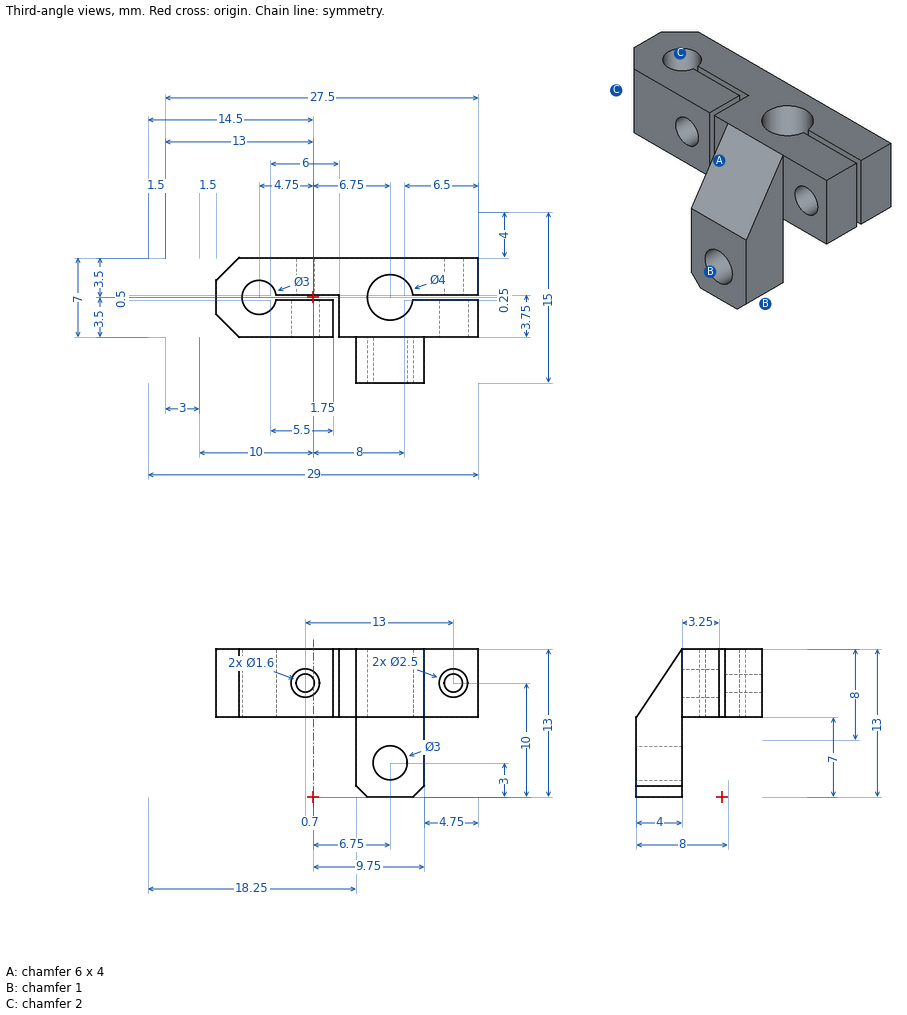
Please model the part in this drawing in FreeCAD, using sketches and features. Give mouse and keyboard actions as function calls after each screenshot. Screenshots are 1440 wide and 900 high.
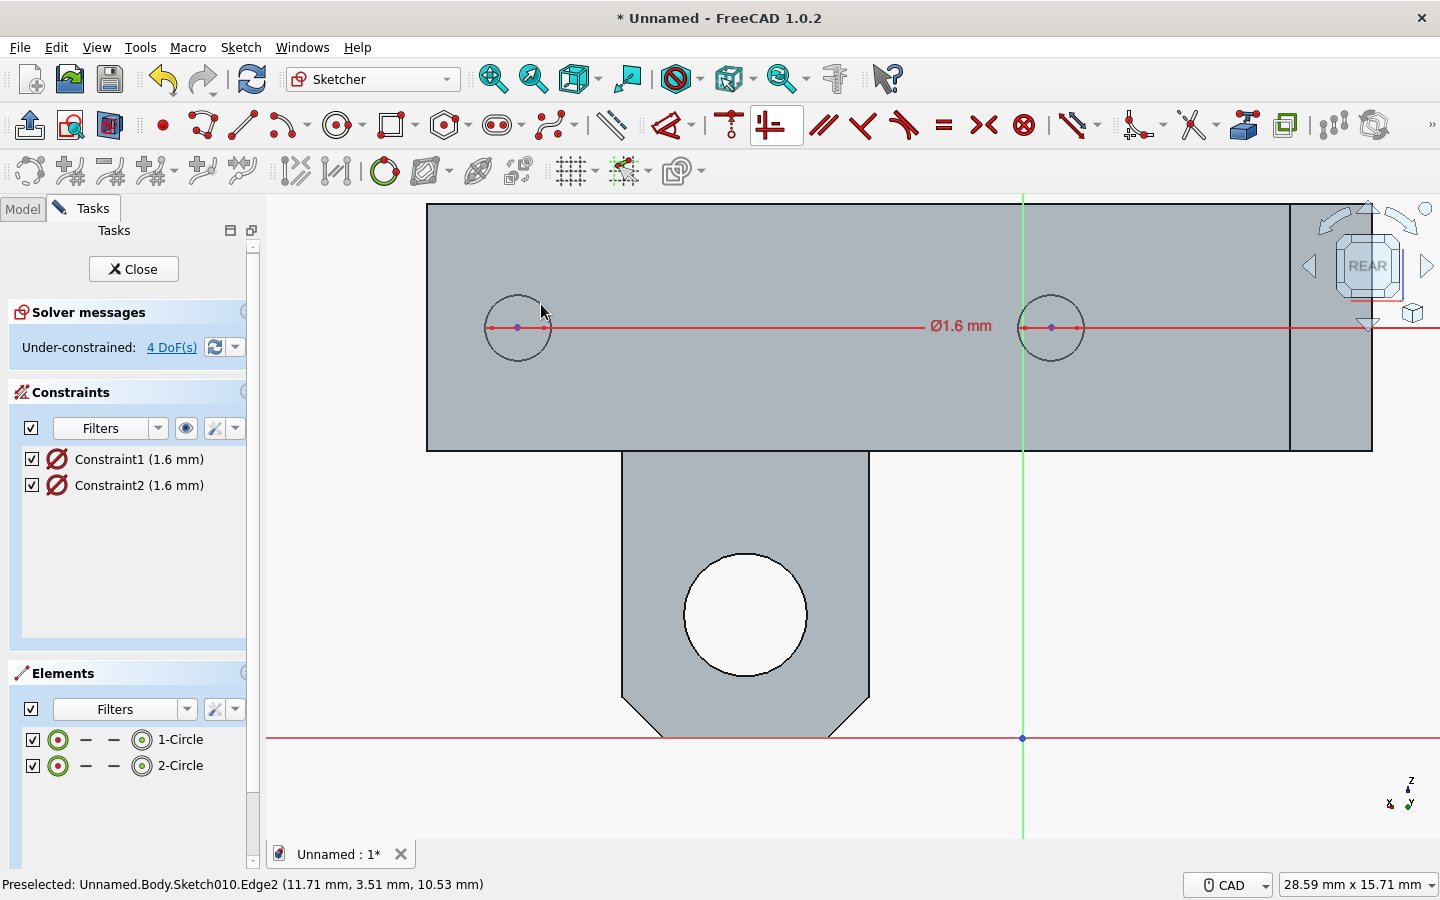
click(1051, 328)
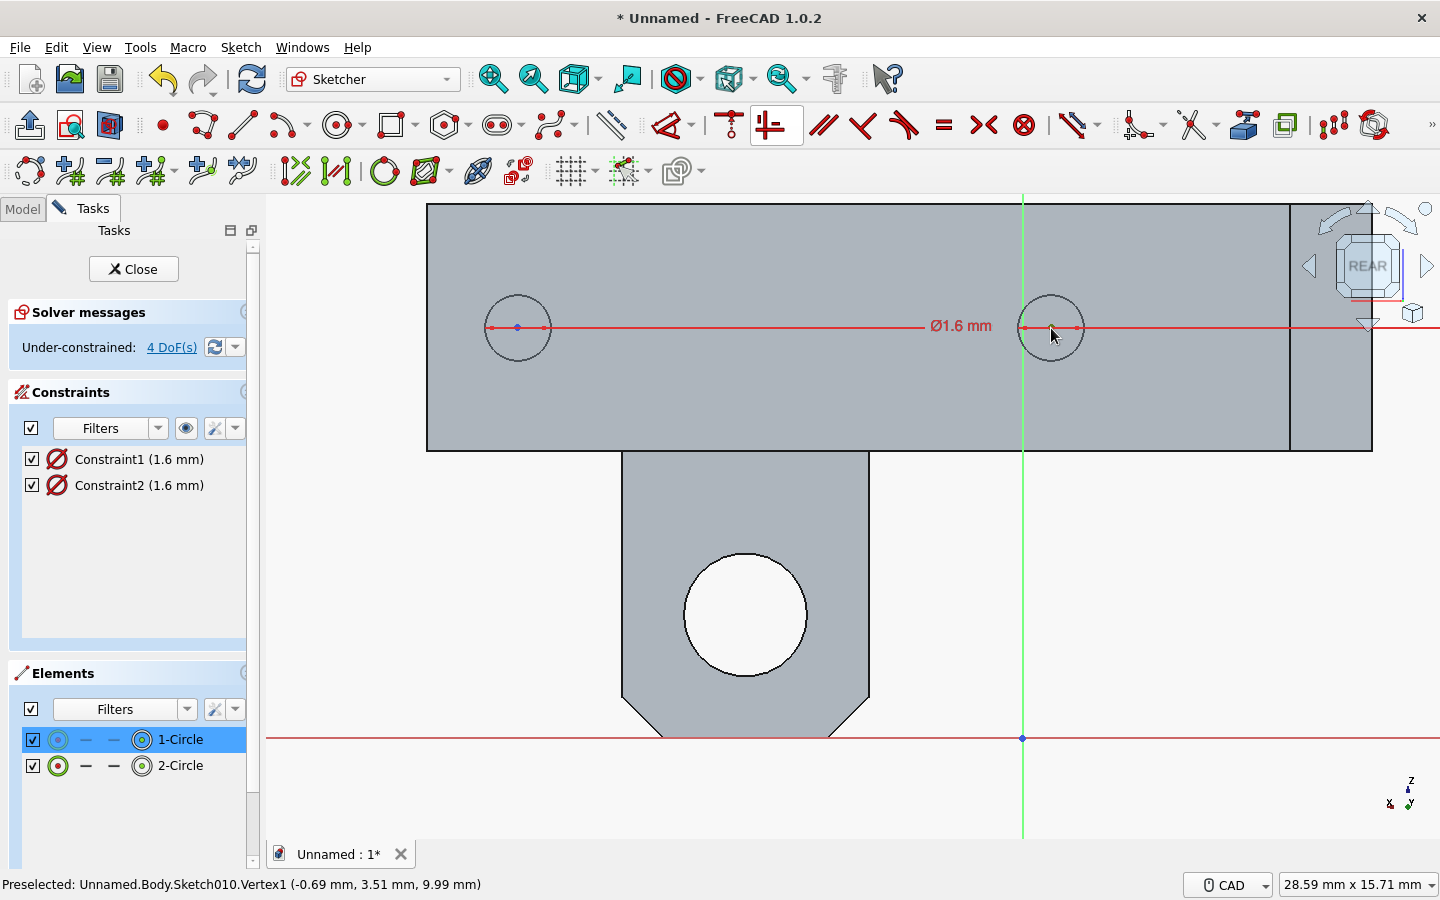
click(518, 328)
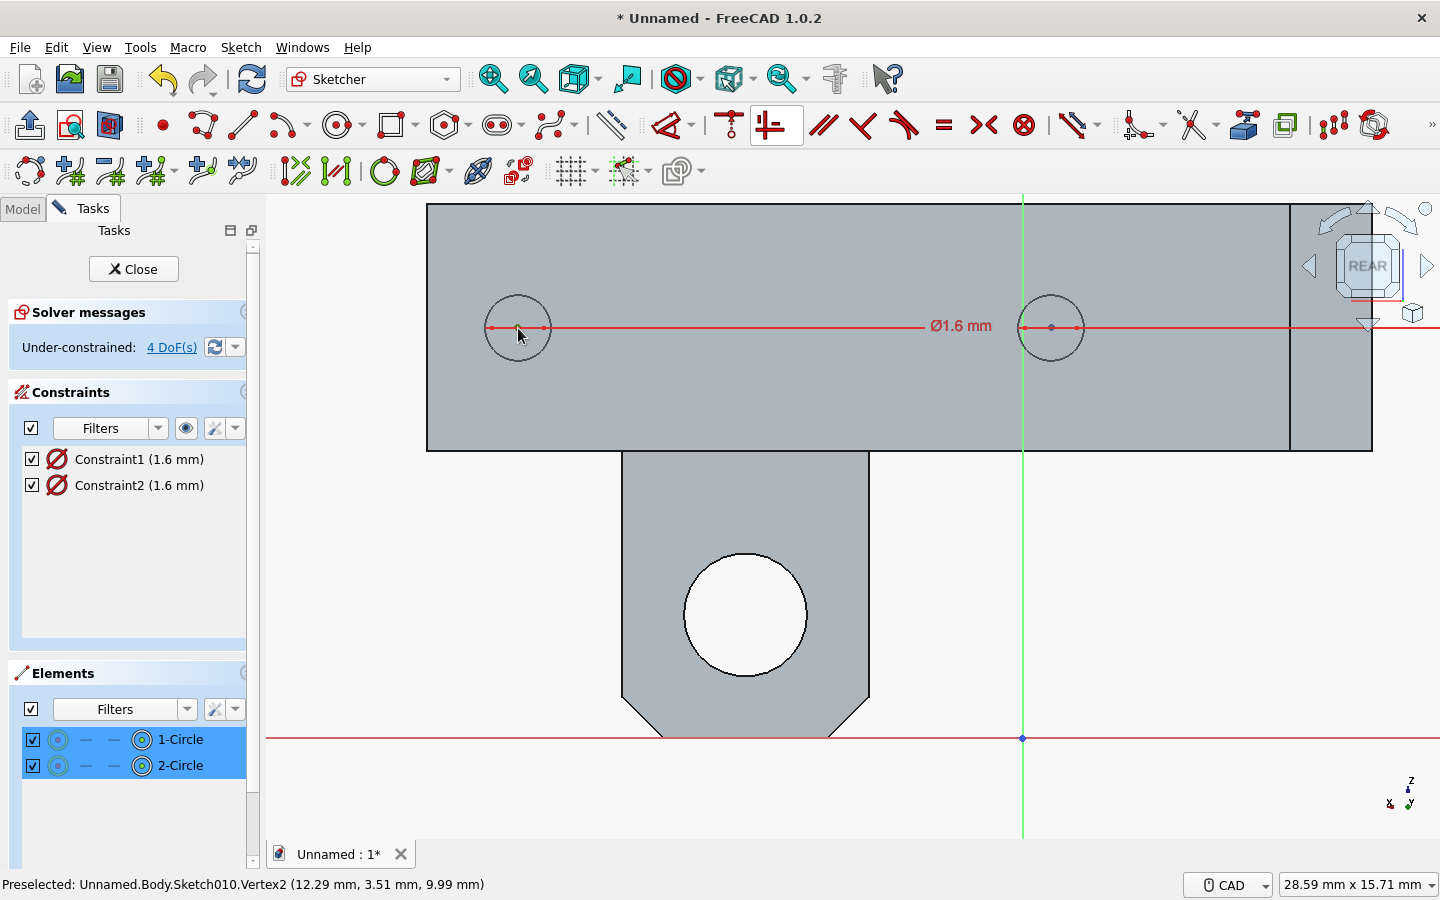
click(798, 126)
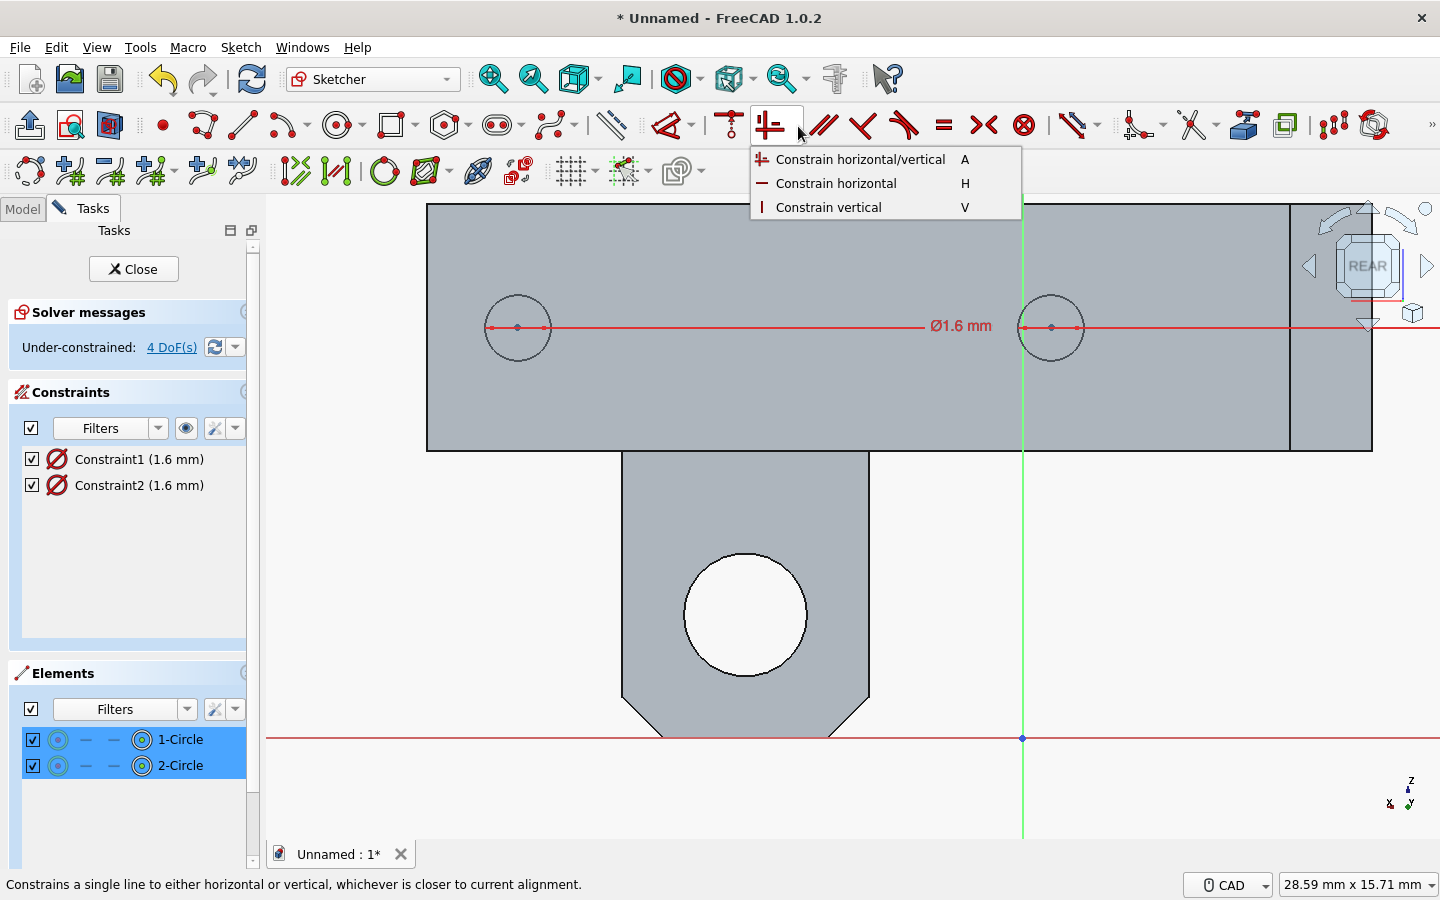
click(886, 183)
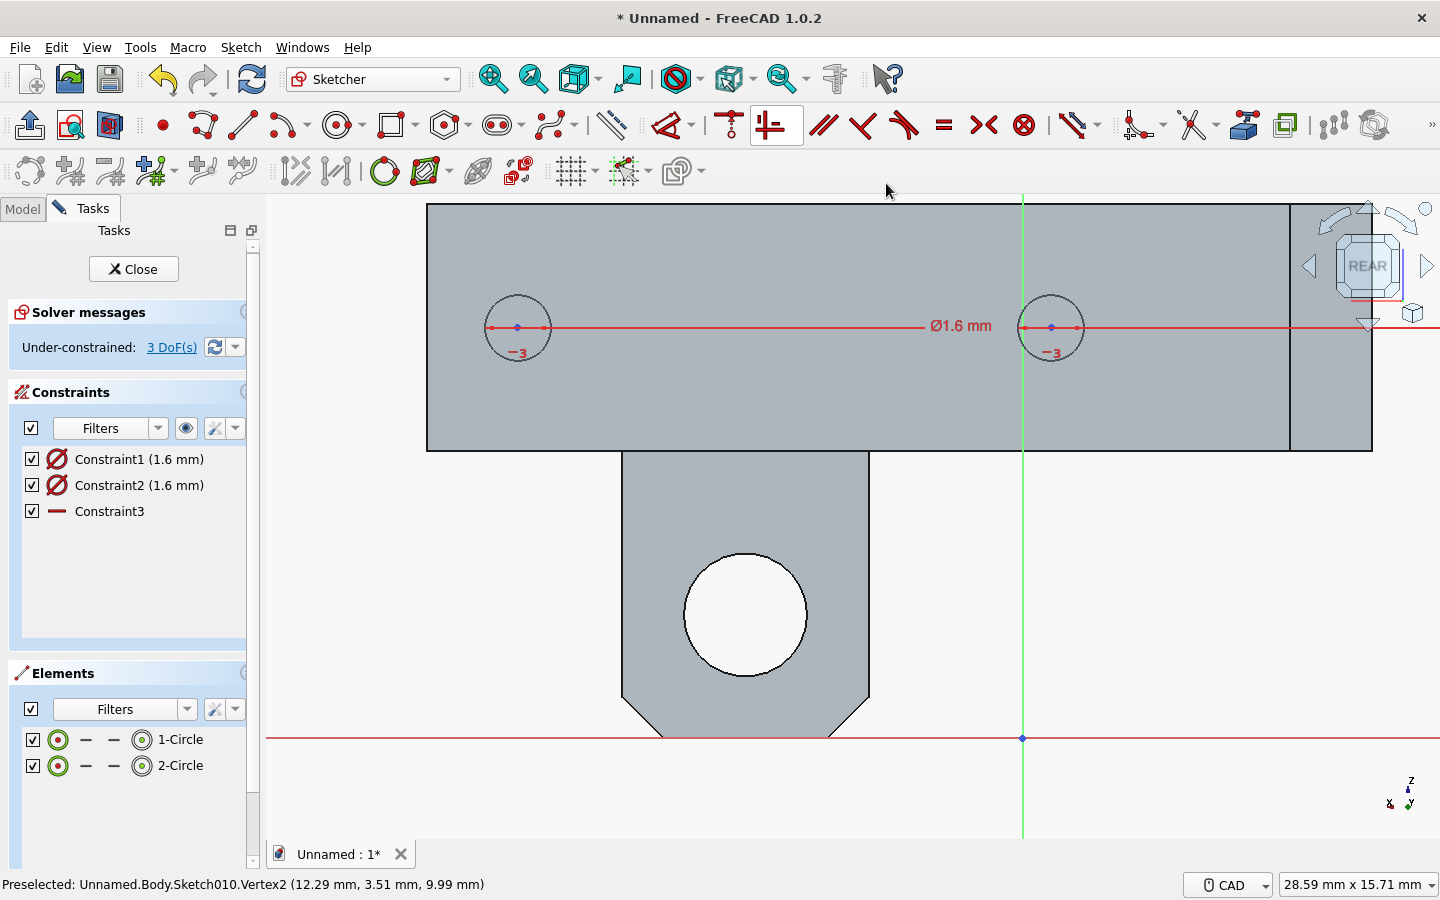
click(666, 126)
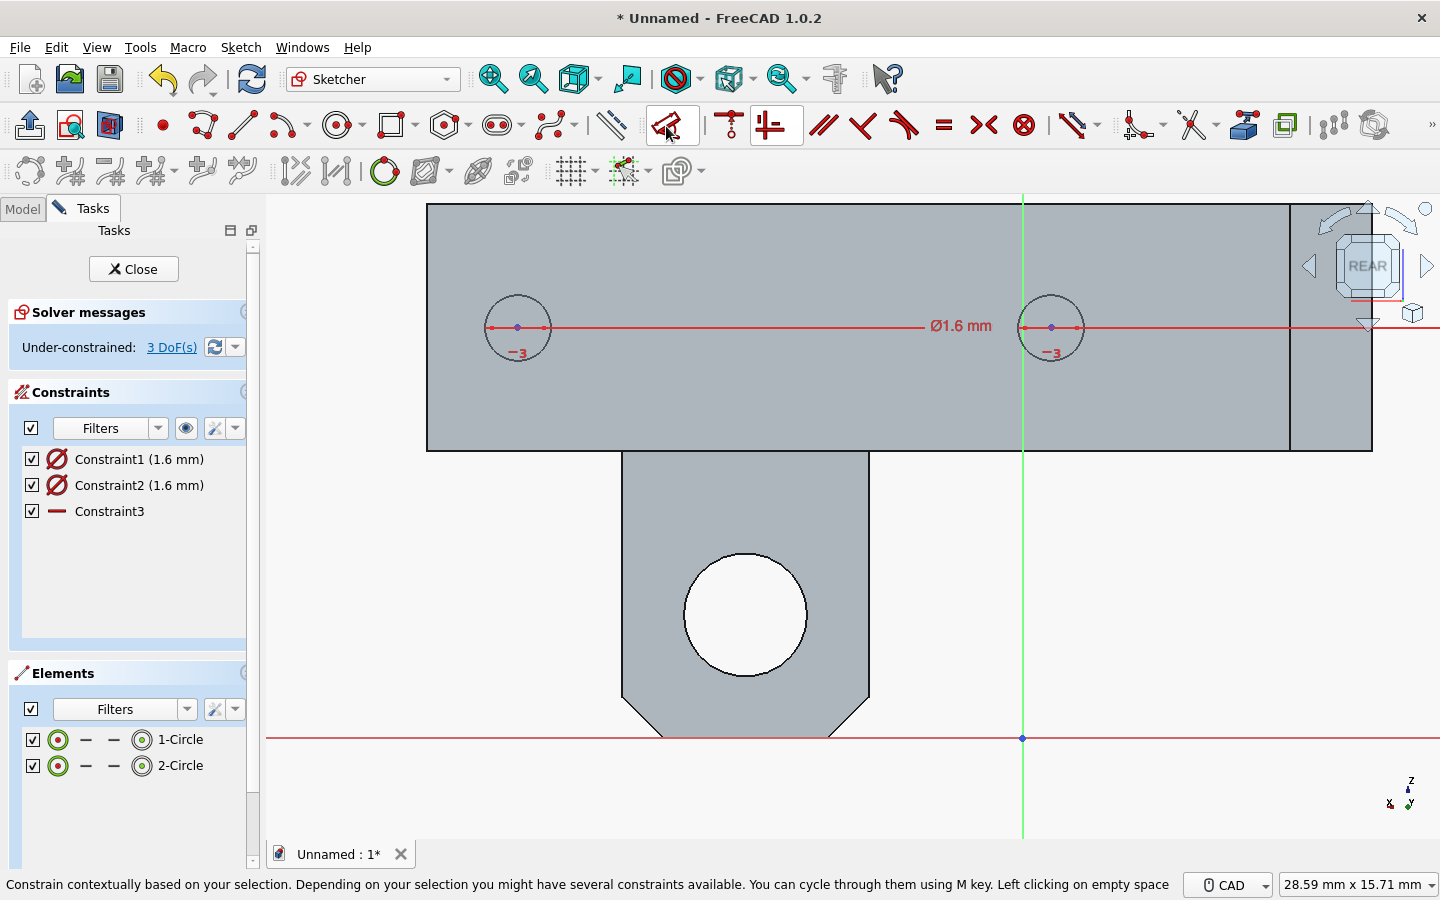
click(1051, 328)
click(1085, 533)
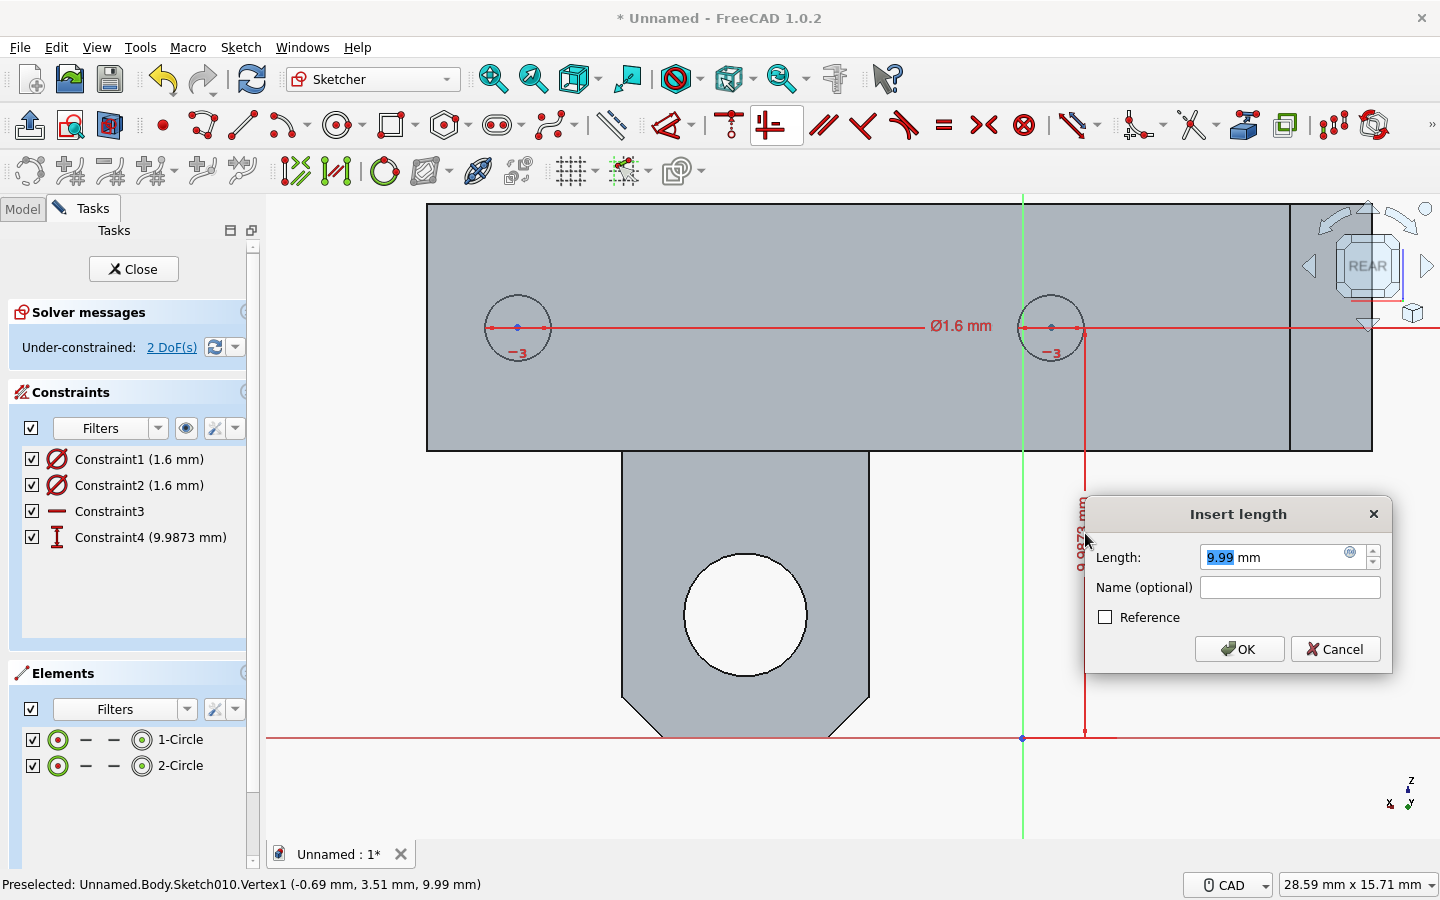
text(10)
key(Return)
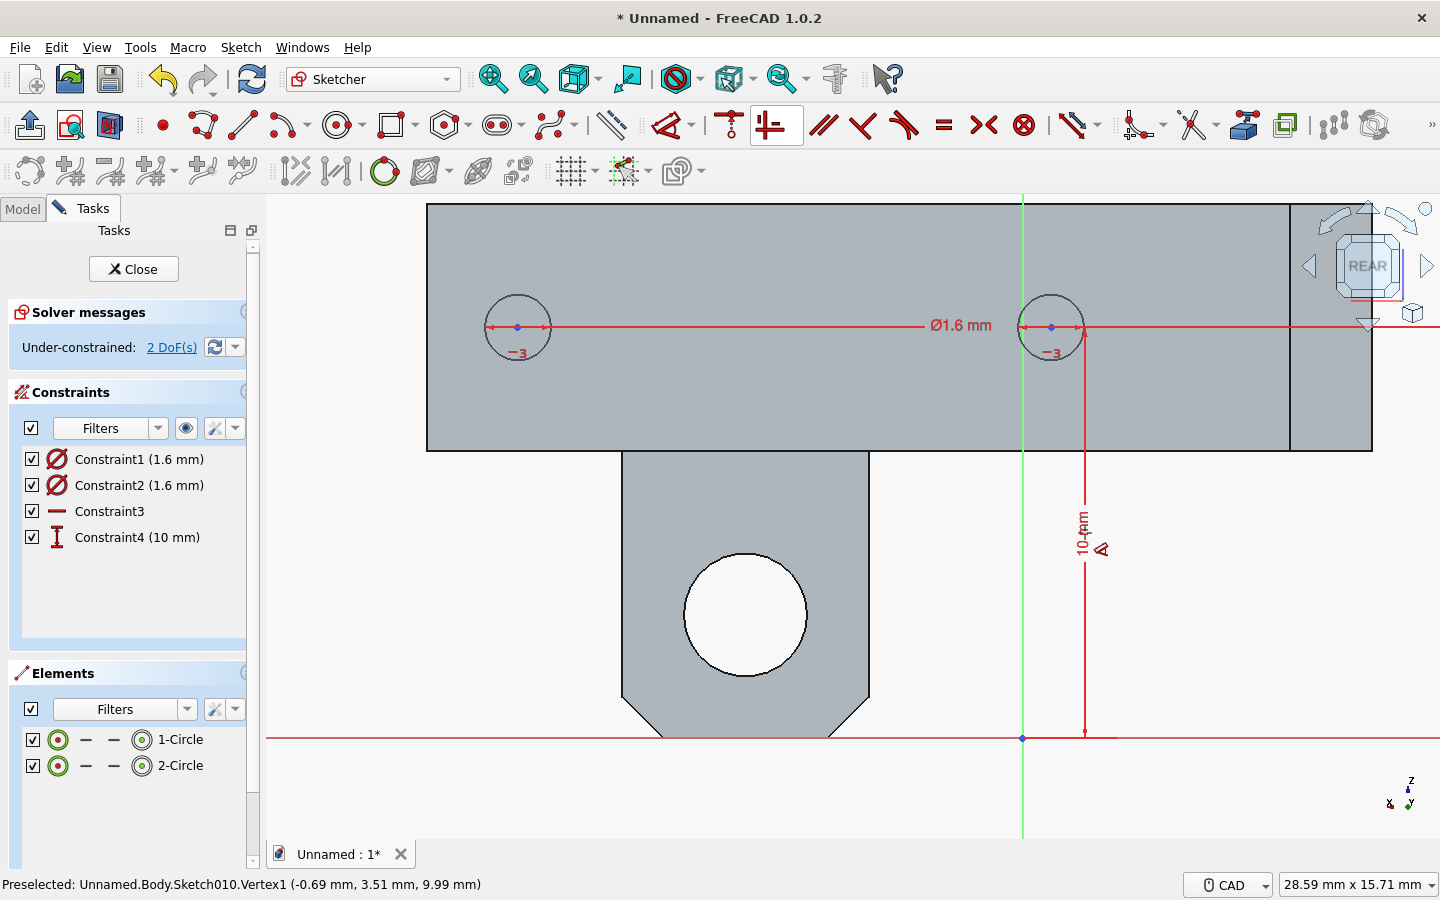
scroll(1051, 327, up, 2)